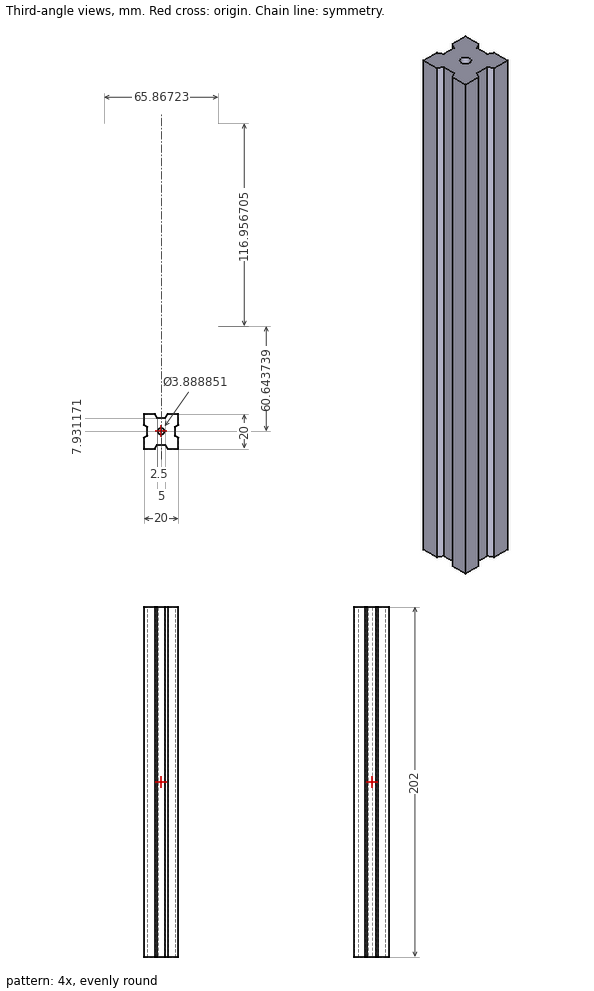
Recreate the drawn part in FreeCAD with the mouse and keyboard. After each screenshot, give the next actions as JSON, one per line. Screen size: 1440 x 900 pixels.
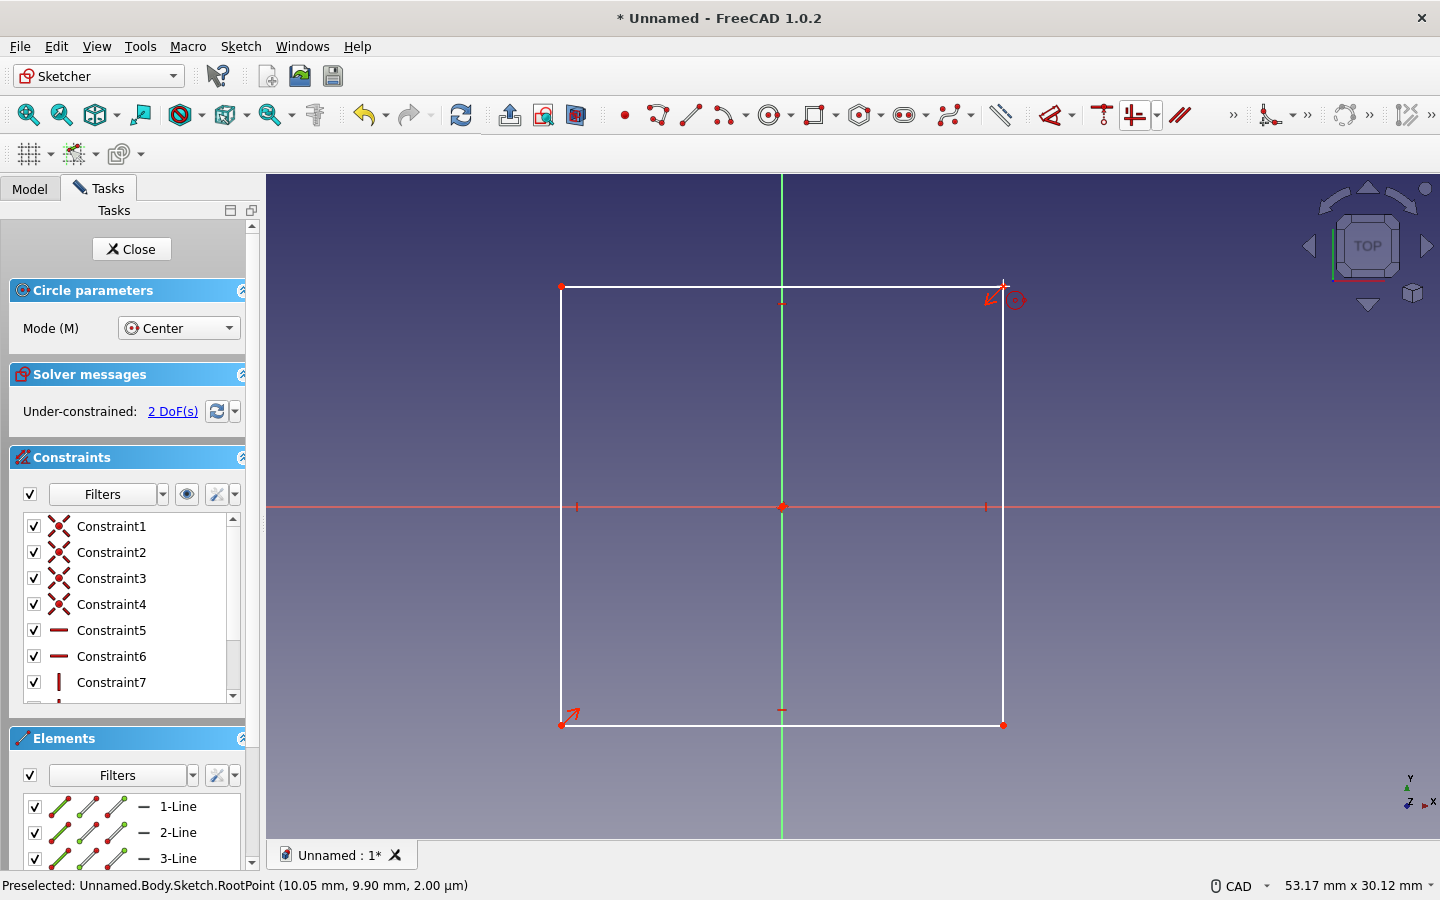
{"action": "left_click", "coordinate": [782, 506]}
{"action": "left_click", "coordinate": [813, 476]}
{"action": "key", "text": "Escape"}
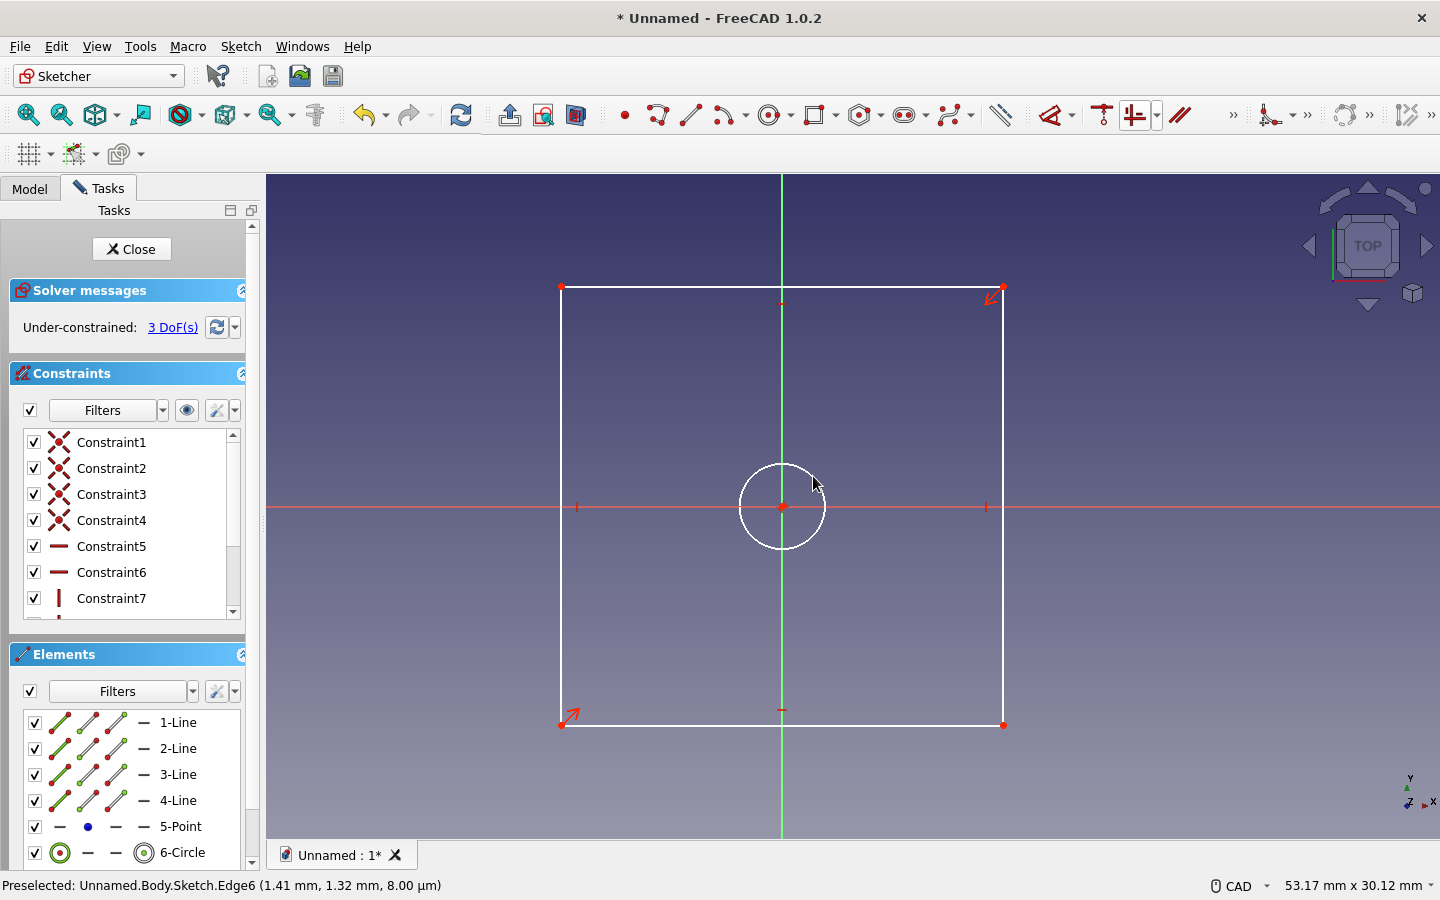
{"action": "left_click", "coordinate": [812, 476]}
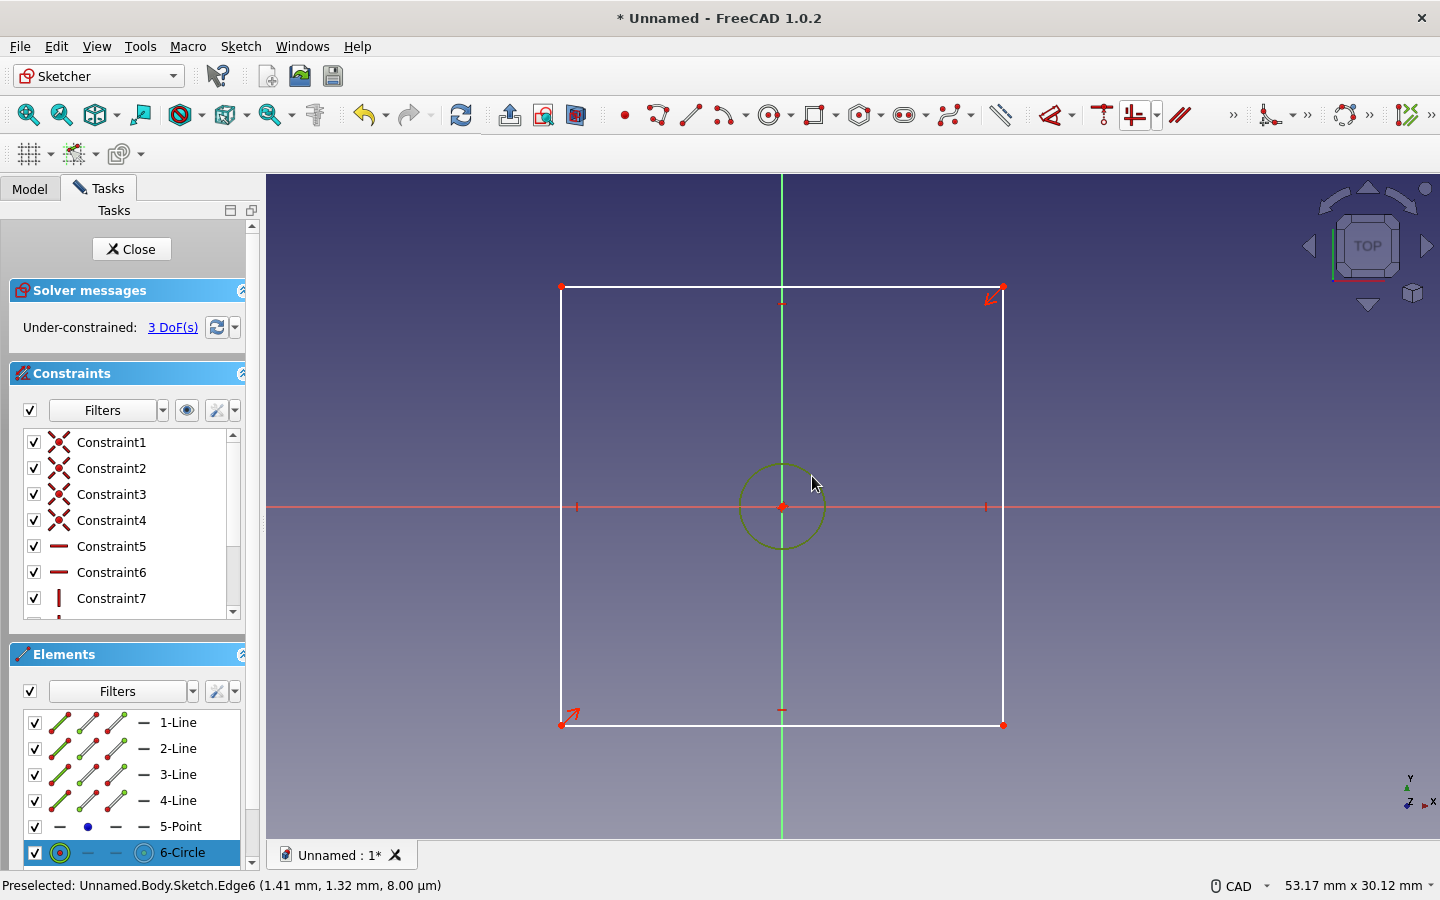
{"action": "key", "text": "k o"}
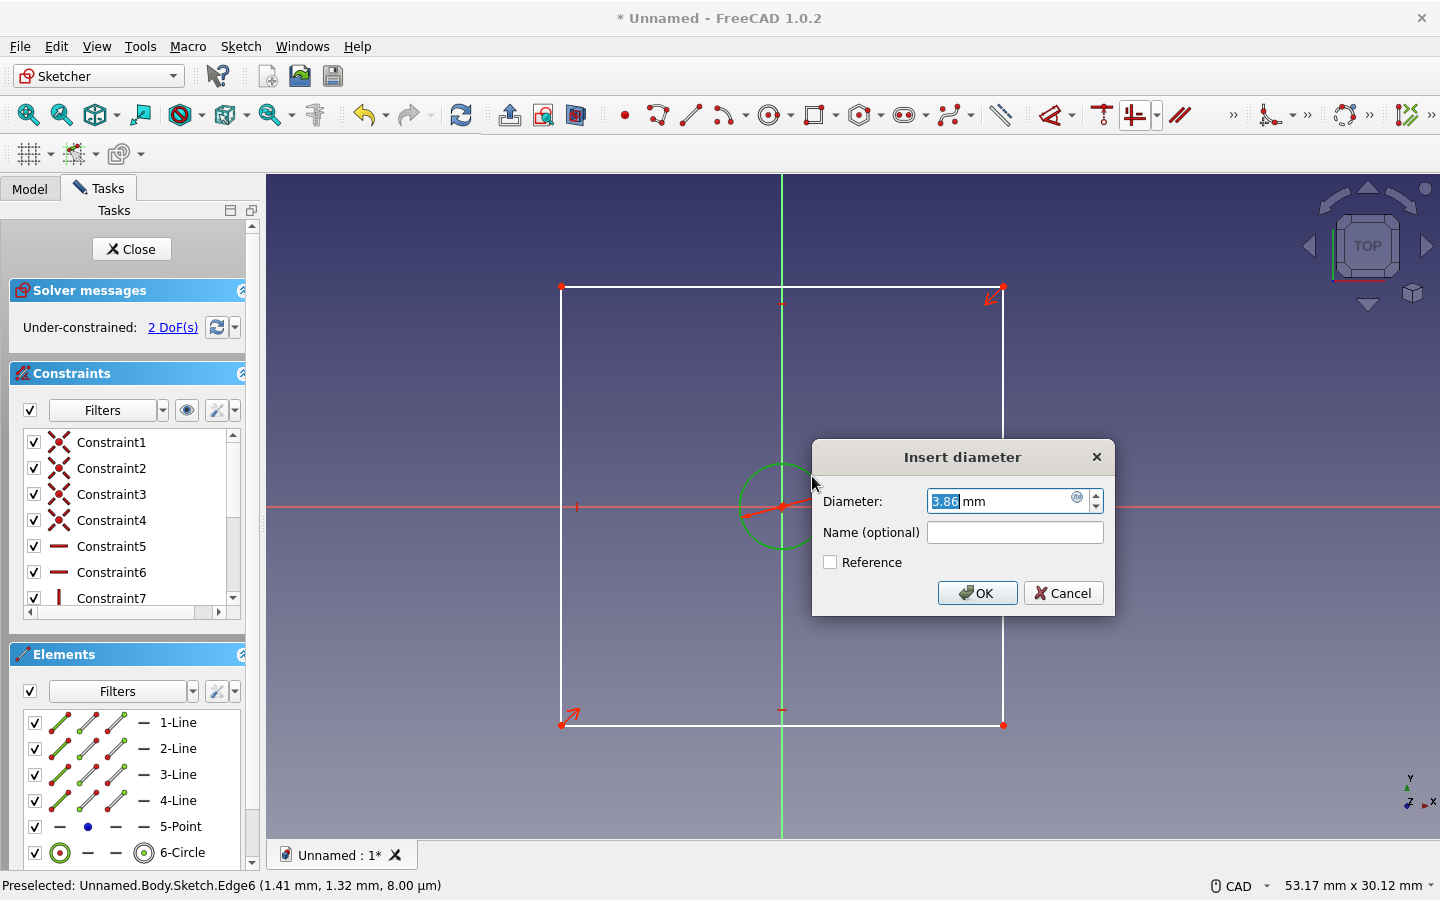
{"action": "type", "text": "3.888851"}
{"action": "key", "text": "Return"}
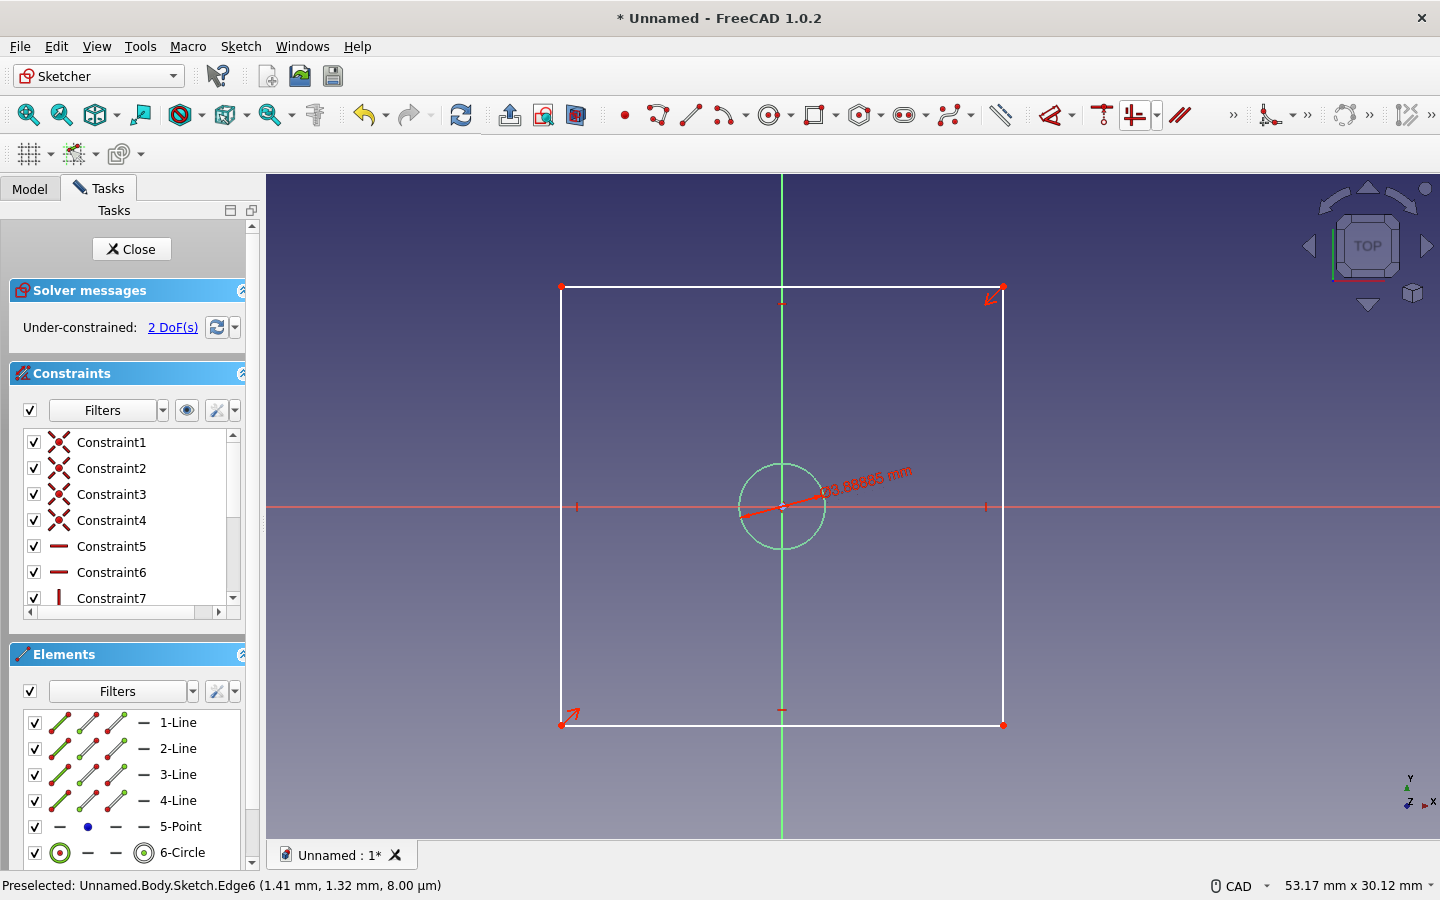
{"action": "left_click", "coordinate": [694, 726]}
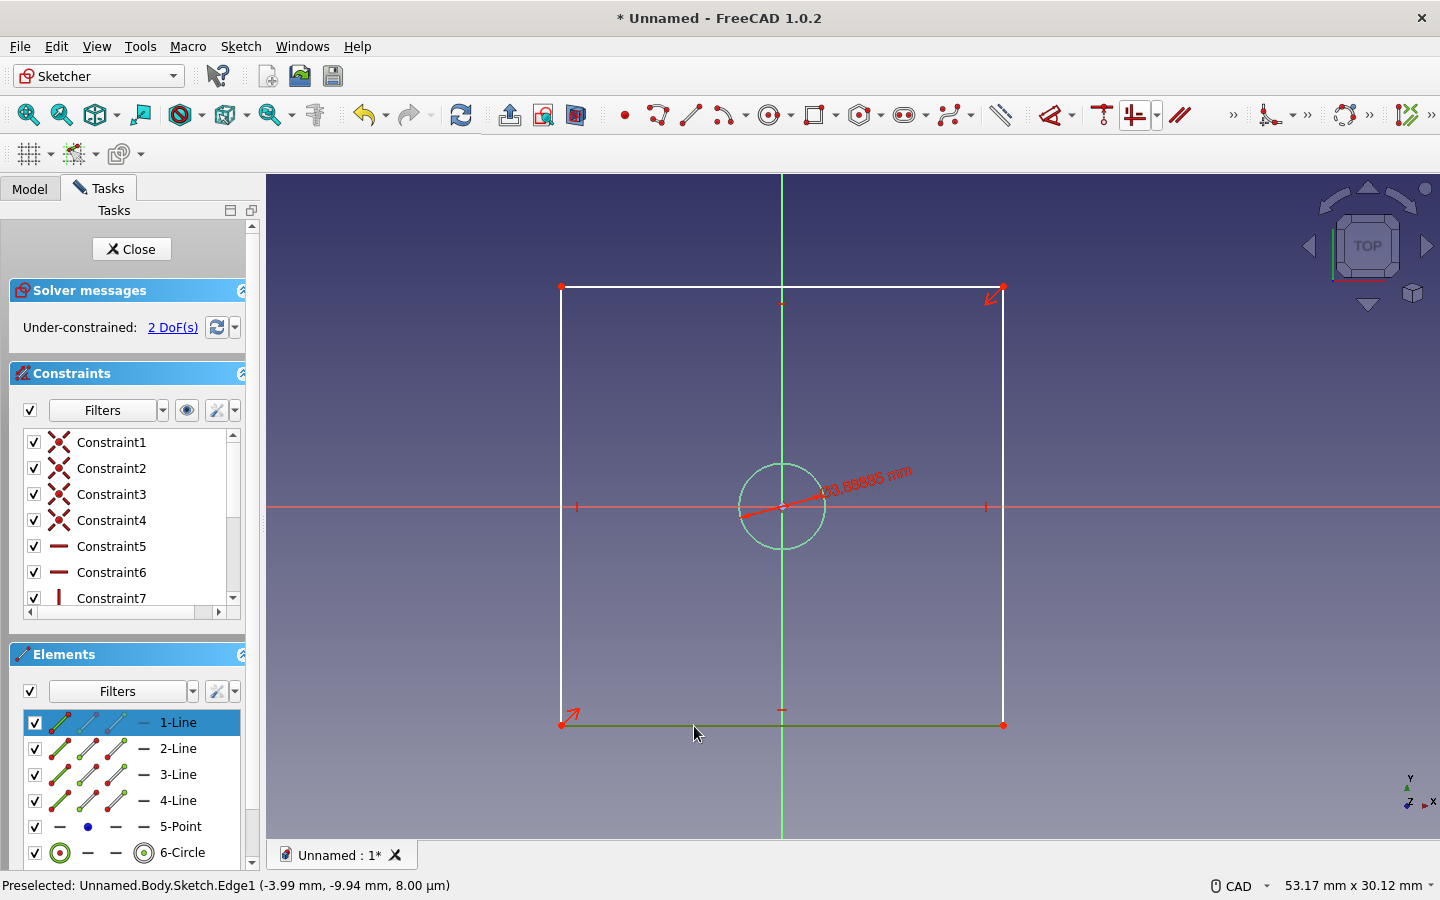
{"action": "key", "text": "l"}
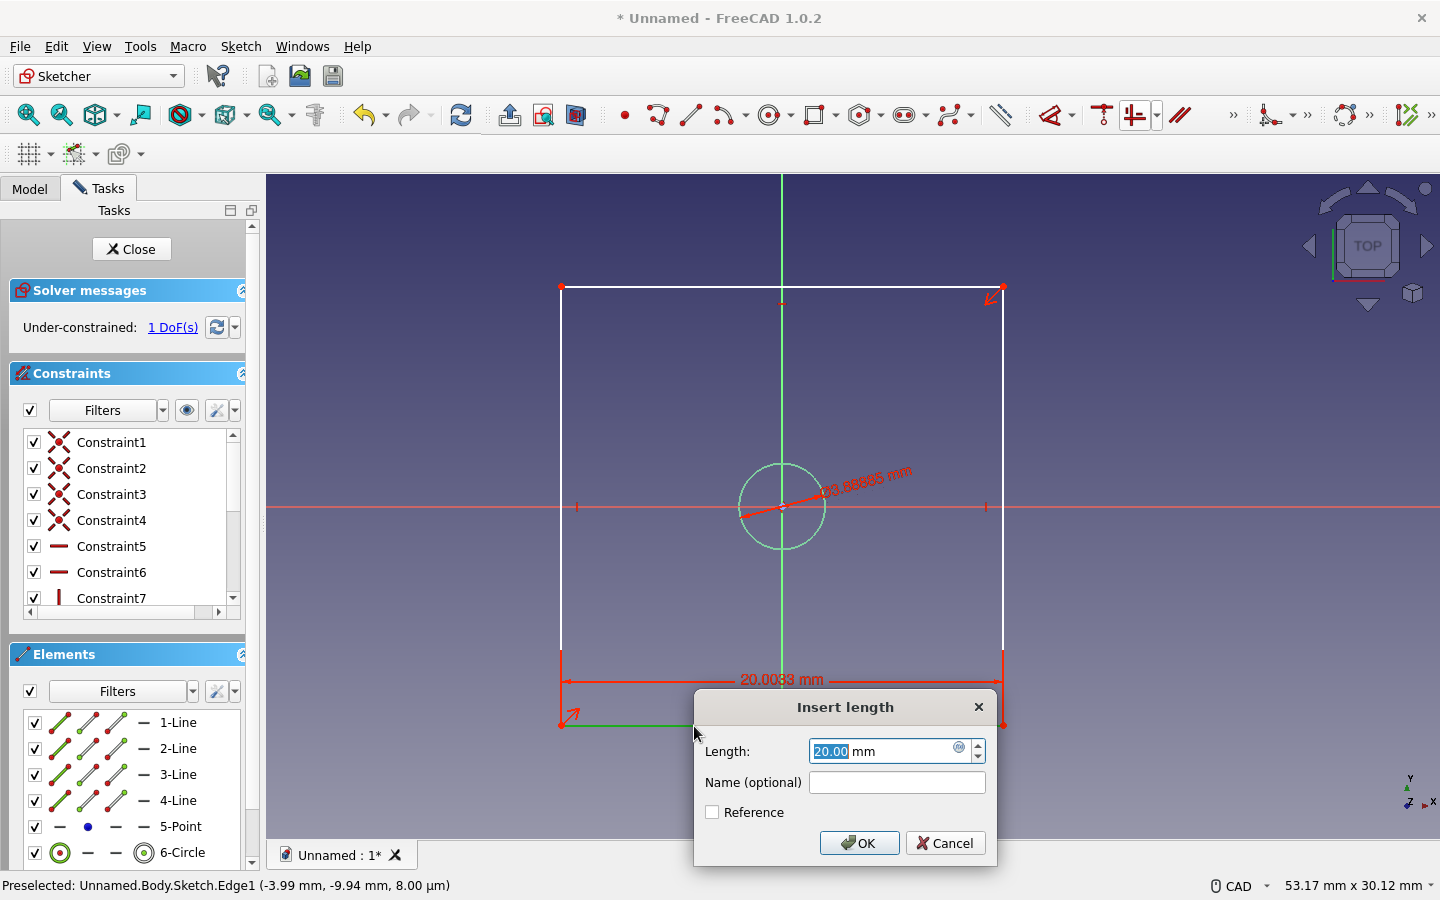
{"action": "type", "text": "20"}
{"action": "key", "text": "Return"}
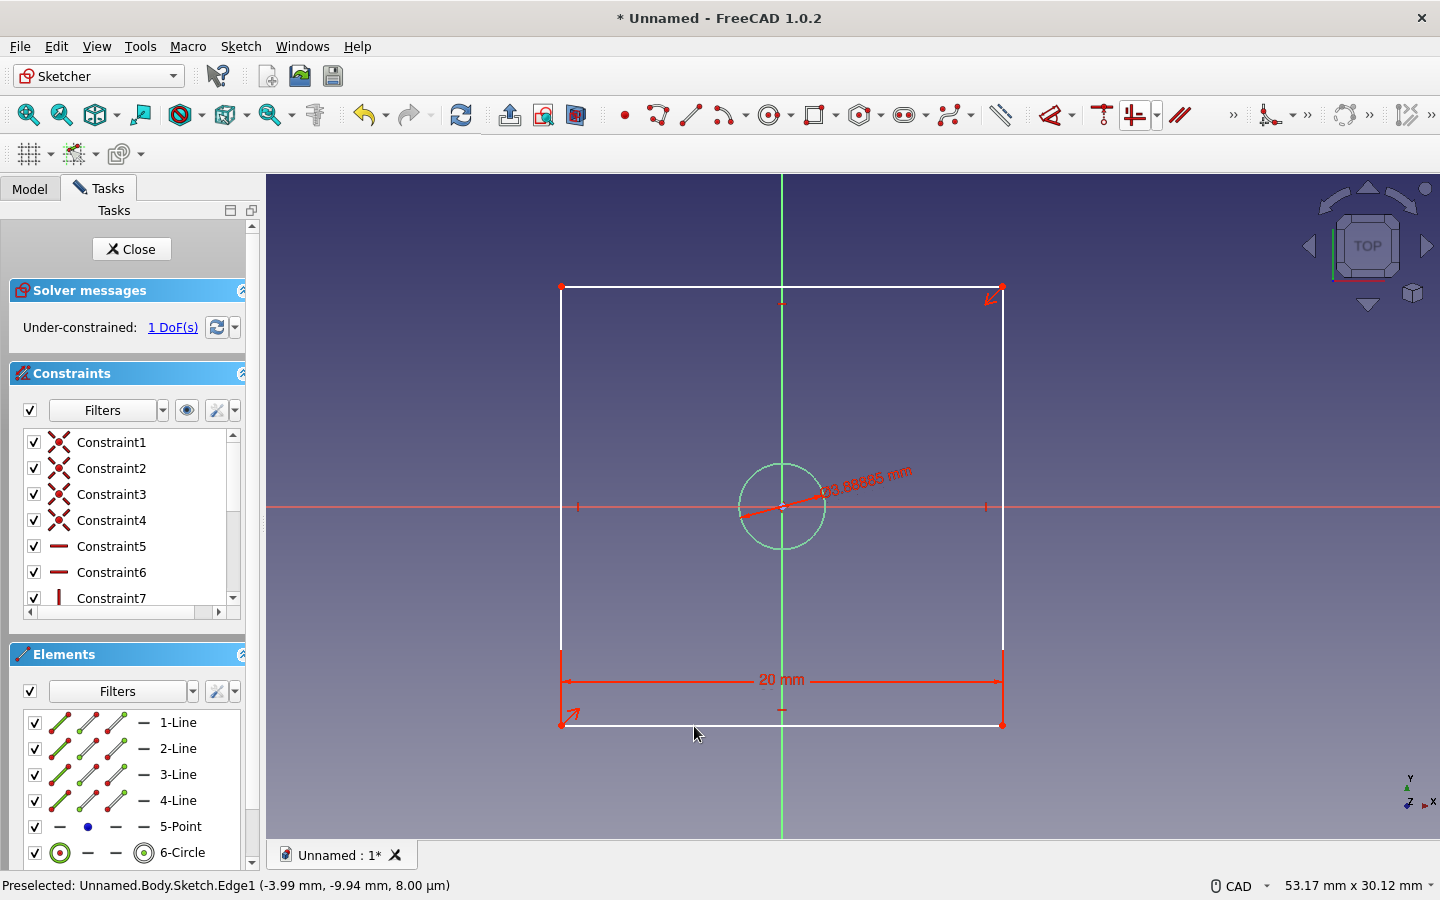
{"action": "left_click", "coordinate": [1003, 594]}